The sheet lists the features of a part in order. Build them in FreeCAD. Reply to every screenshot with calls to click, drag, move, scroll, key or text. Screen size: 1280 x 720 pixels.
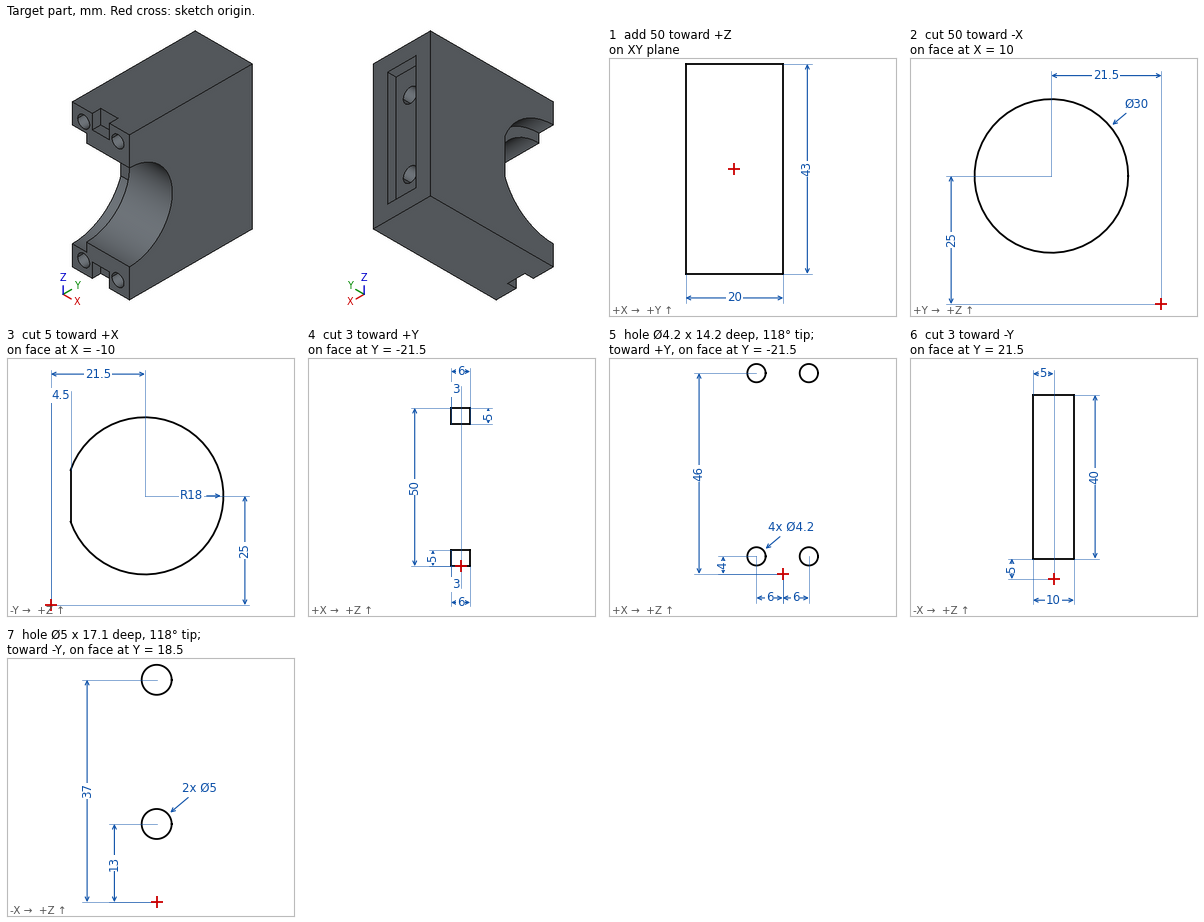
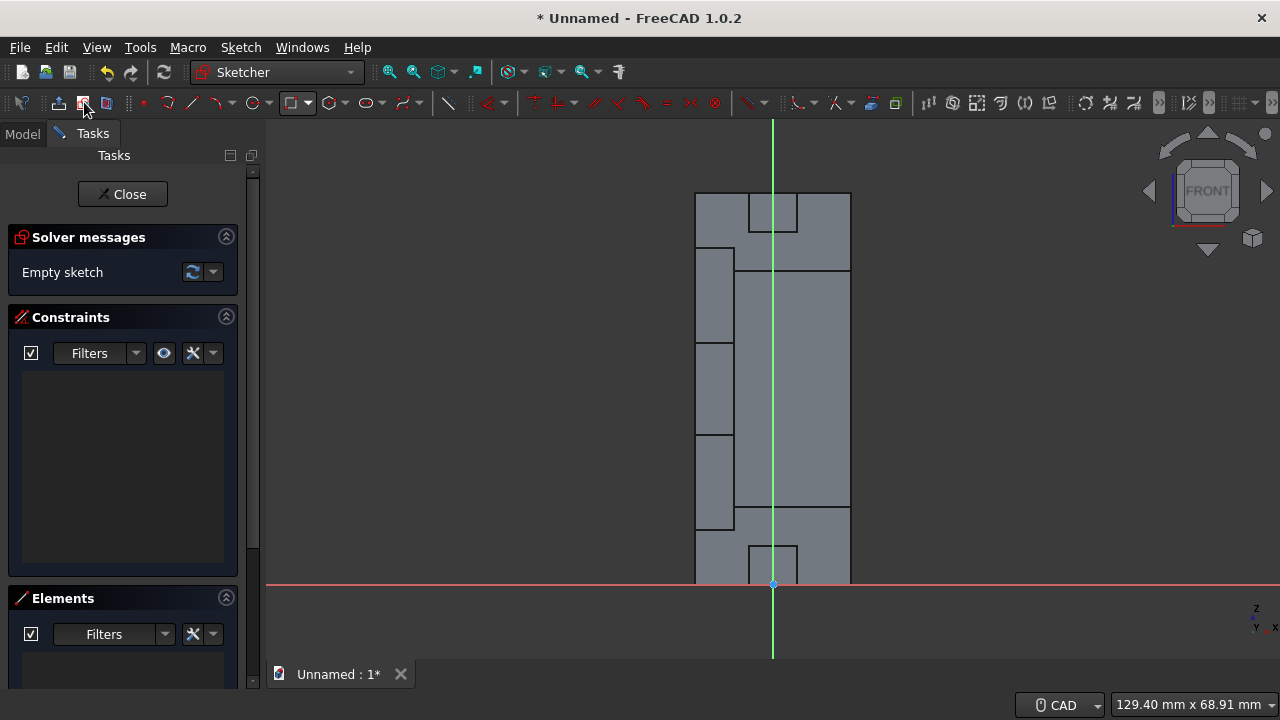
click(254, 104)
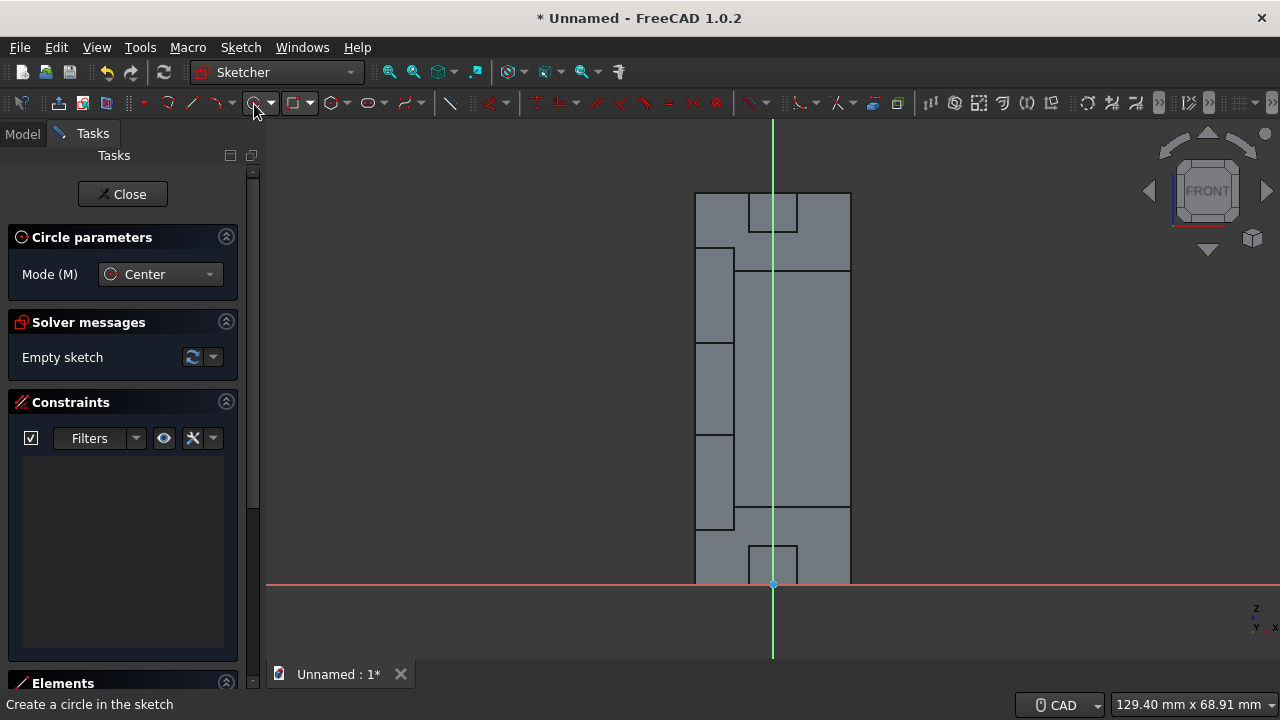
scroll(726, 554, up, 2)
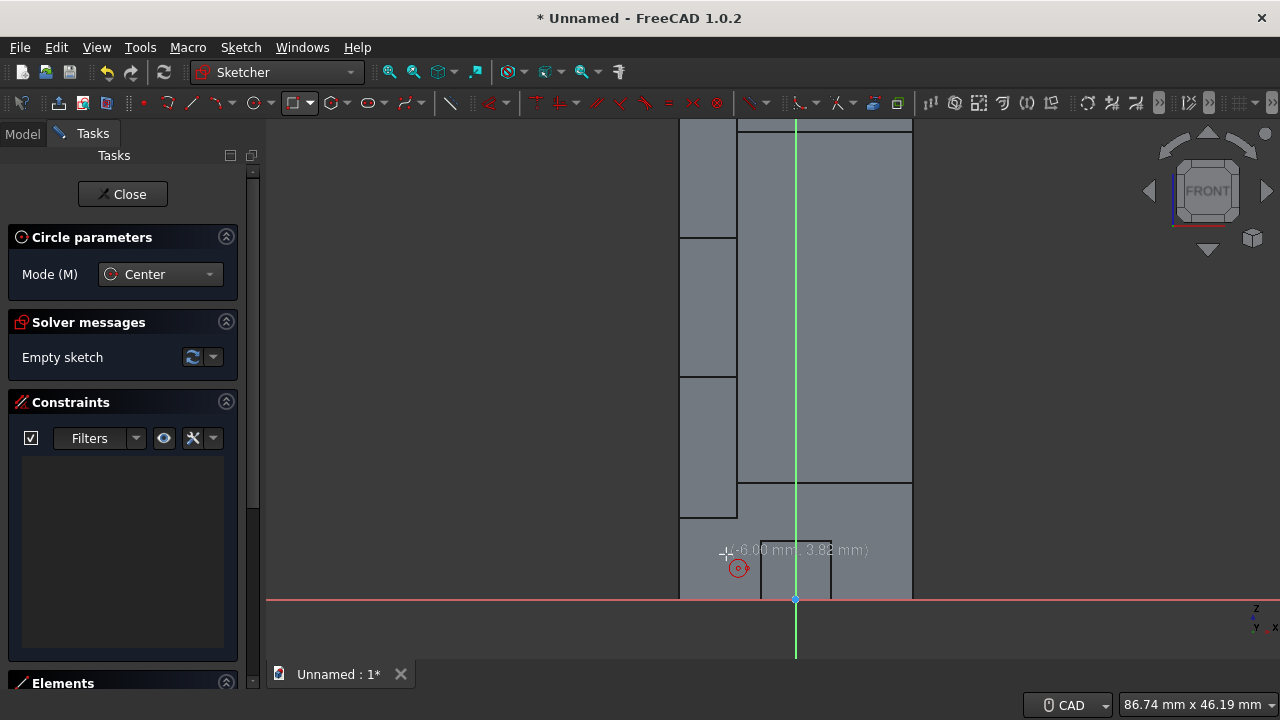
click(726, 553)
move(743, 536)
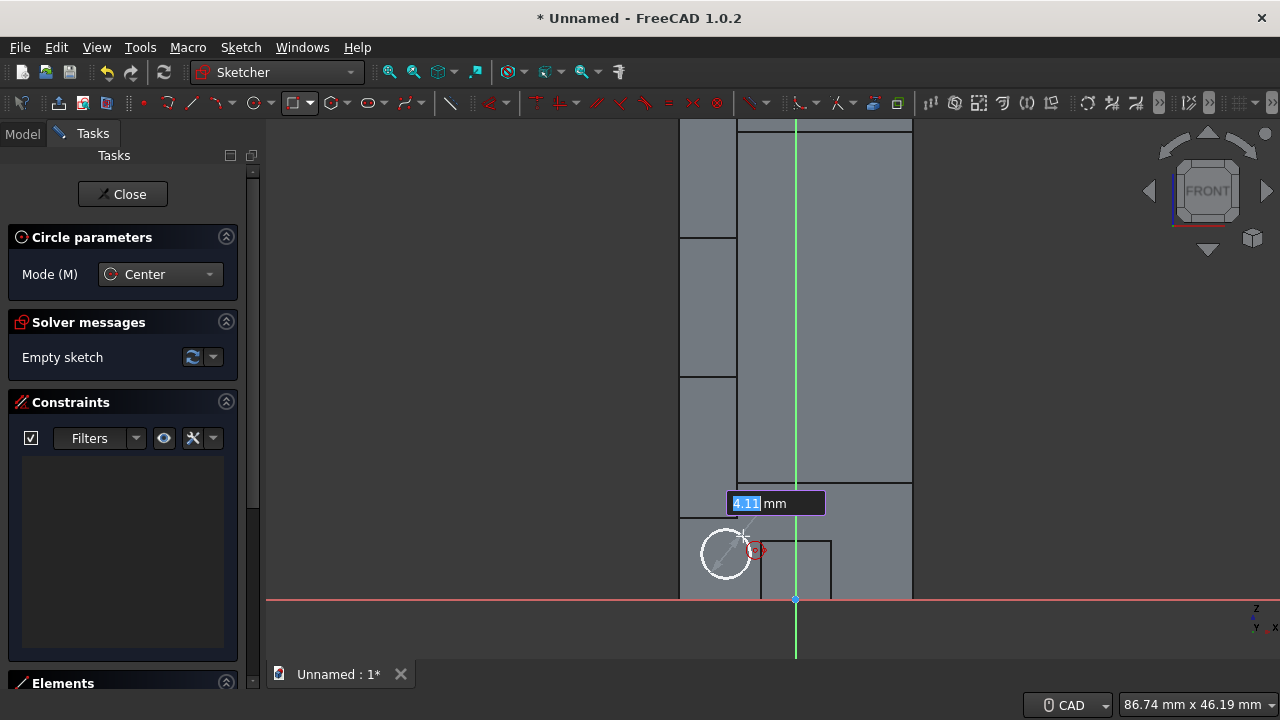
text(4.2)
key(Return)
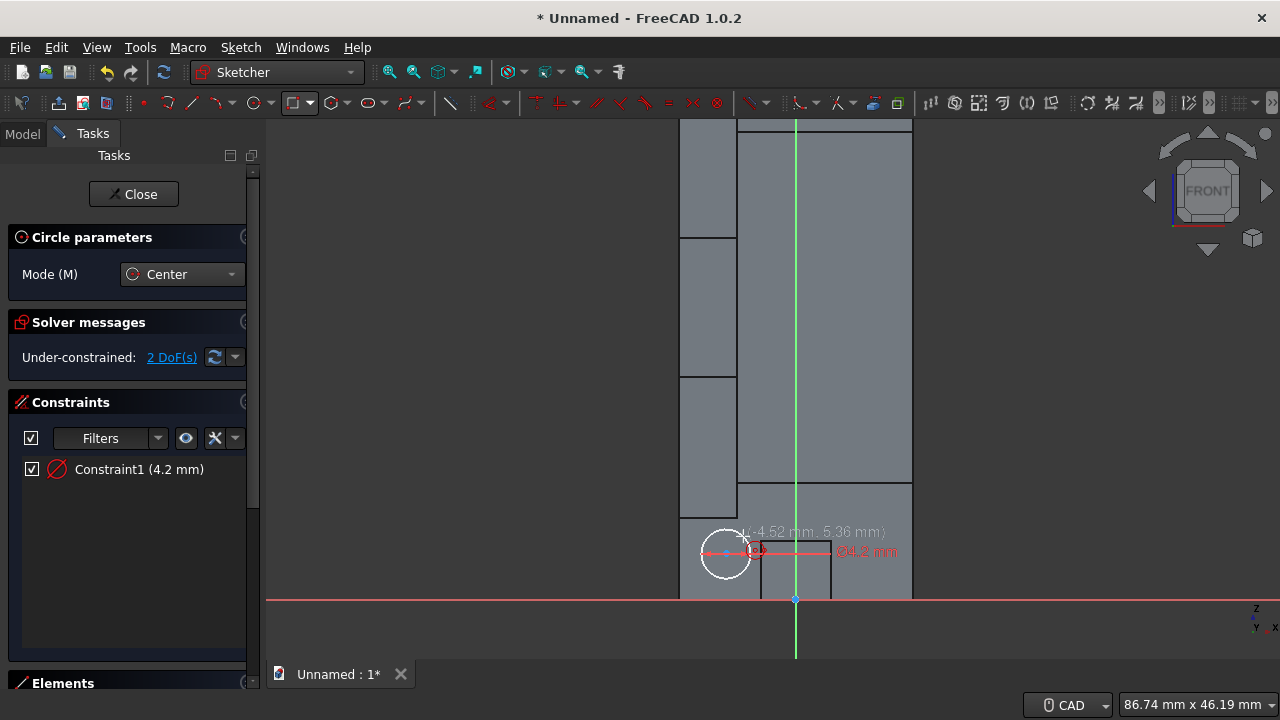
click(866, 553)
move(883, 536)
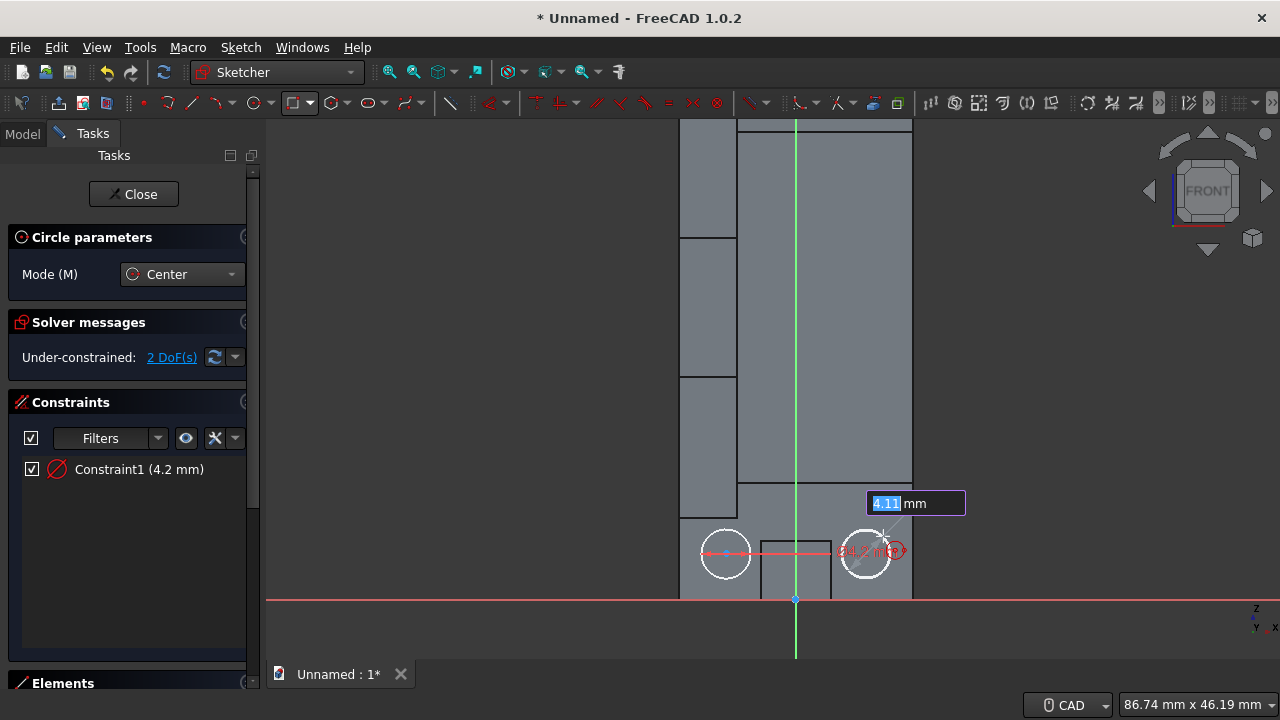
text(4.2)
key(Return)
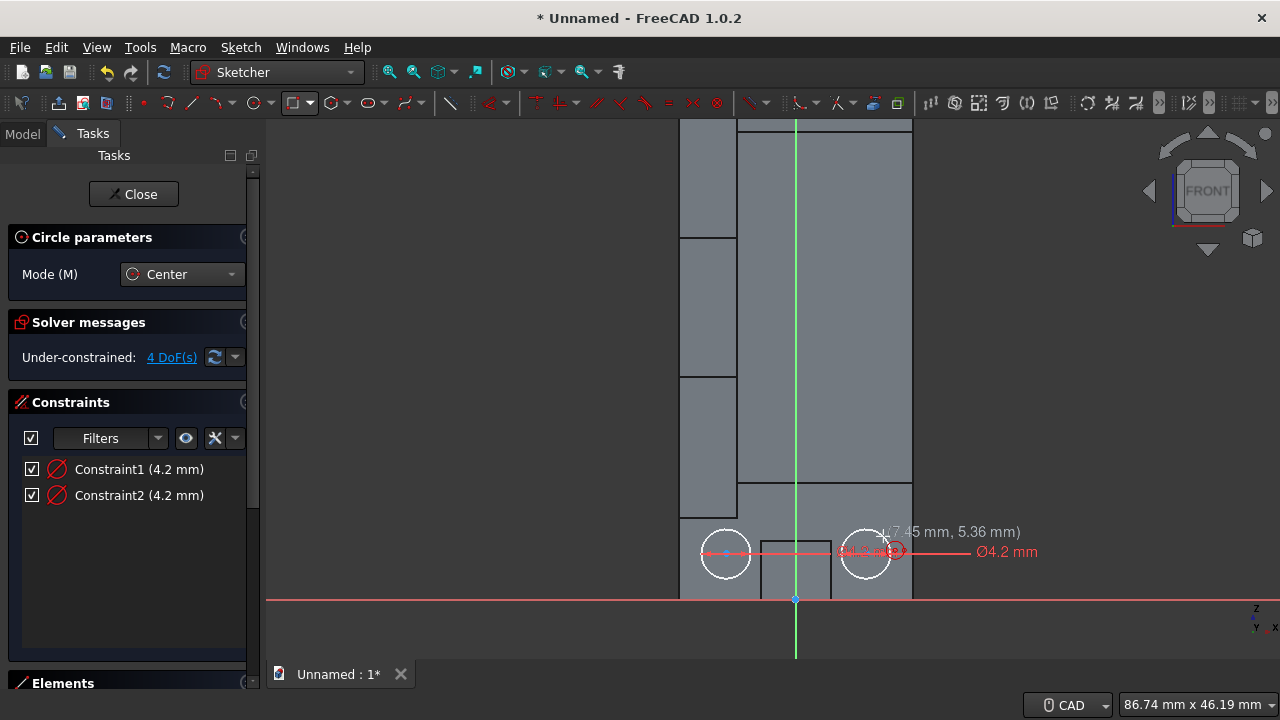
scroll(519, 532, down, 2)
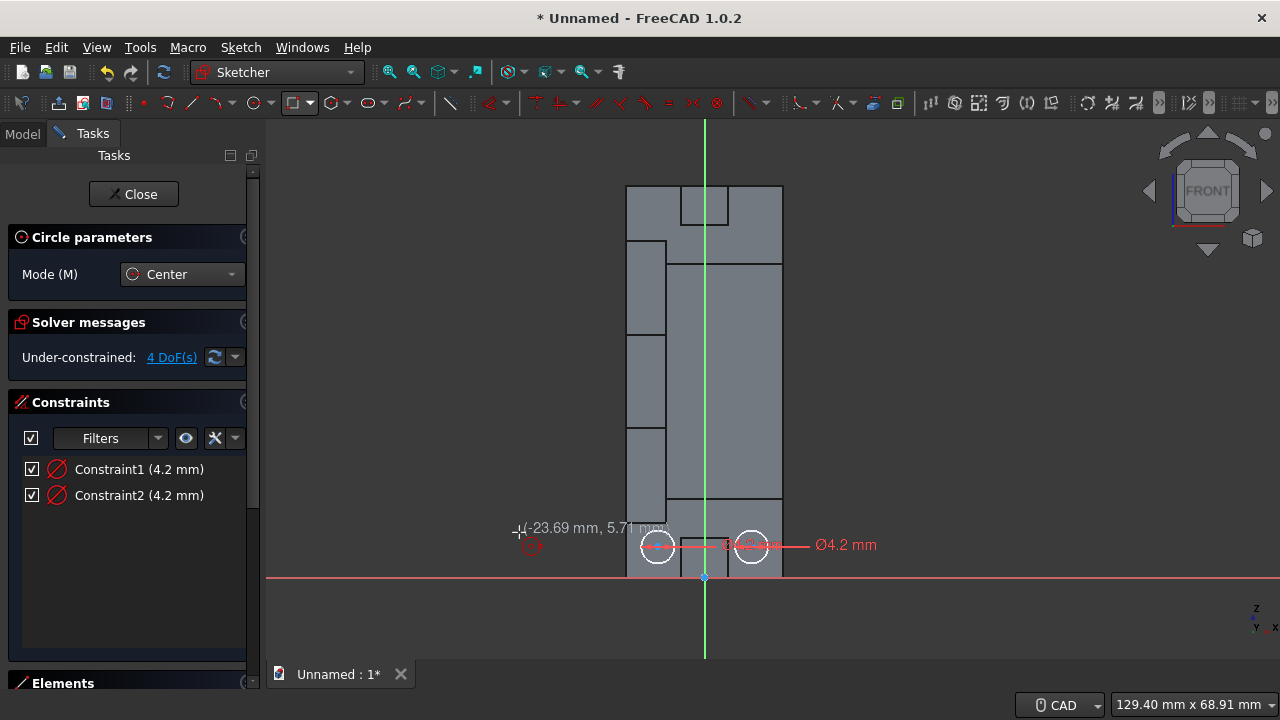
scroll(658, 217, up, 2)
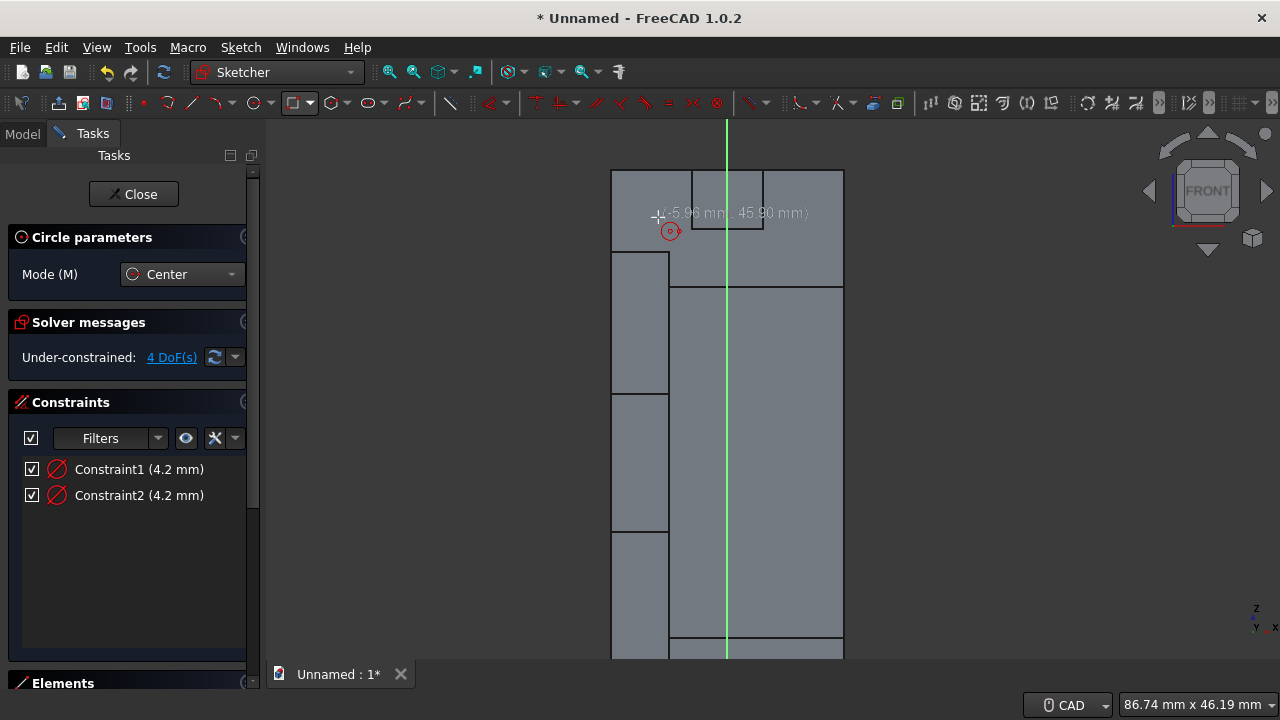
click(657, 217)
move(675, 200)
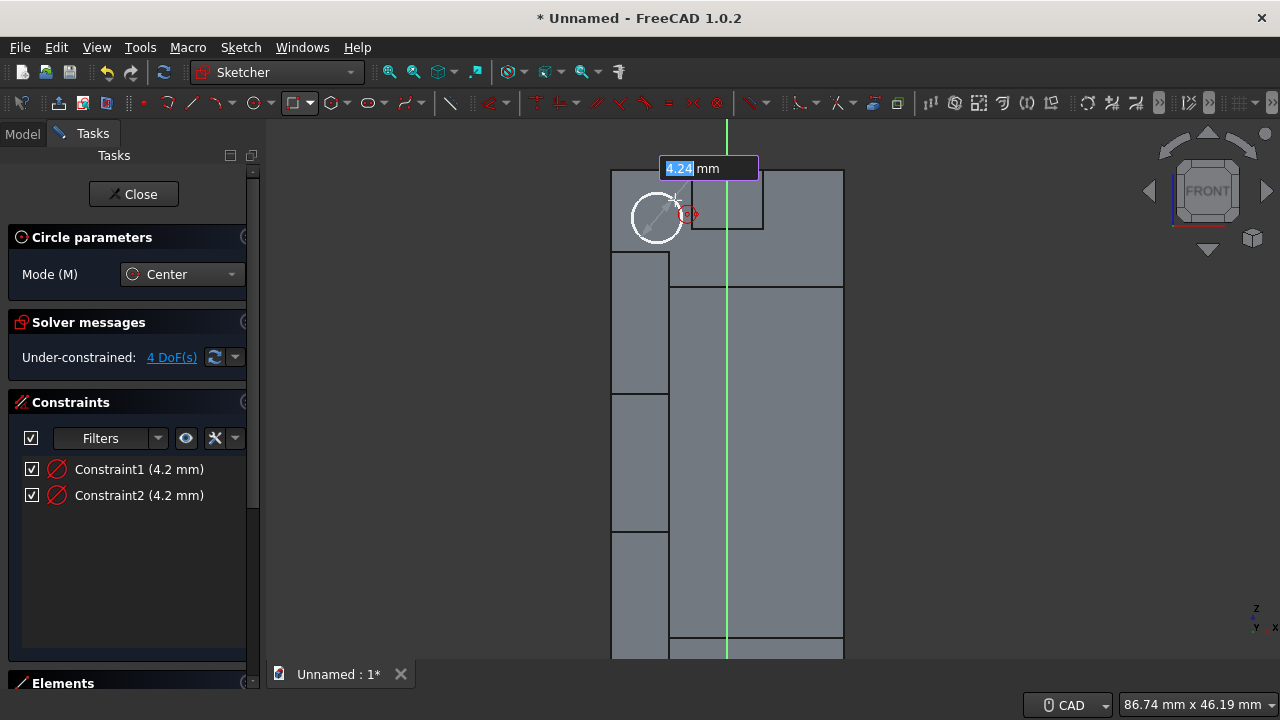
text(4.2)
key(Return)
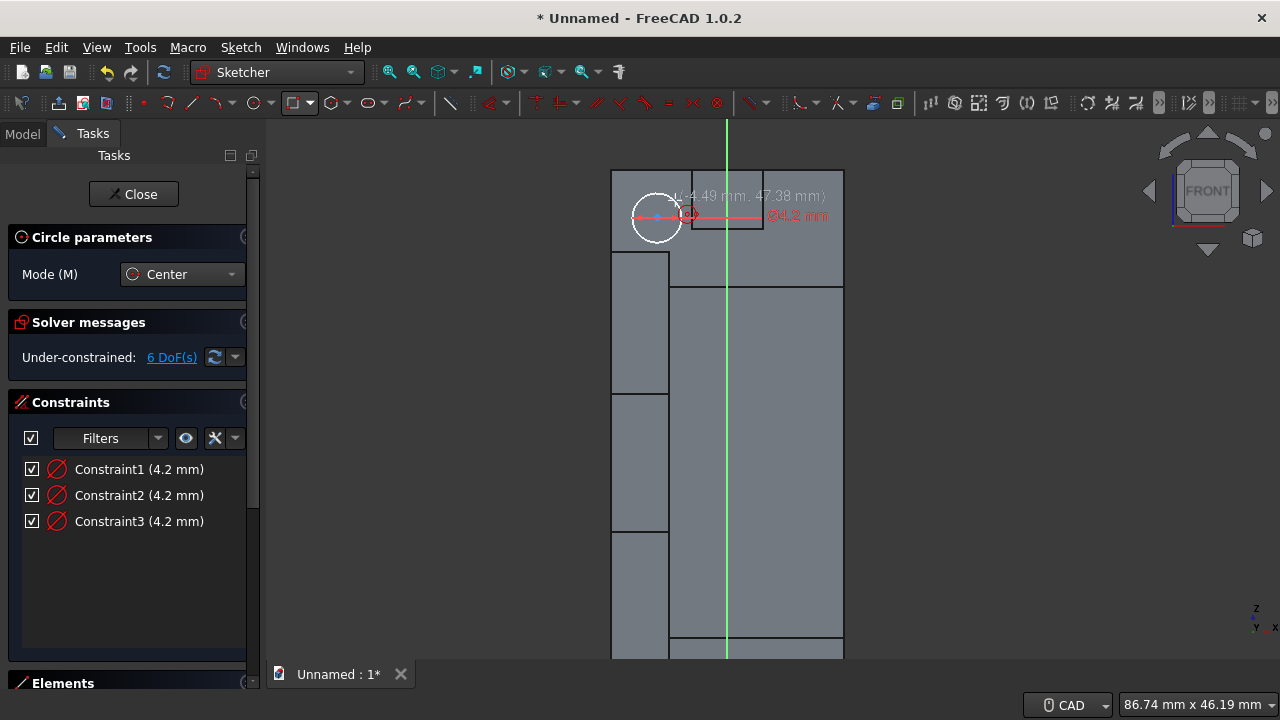
click(798, 217)
move(815, 200)